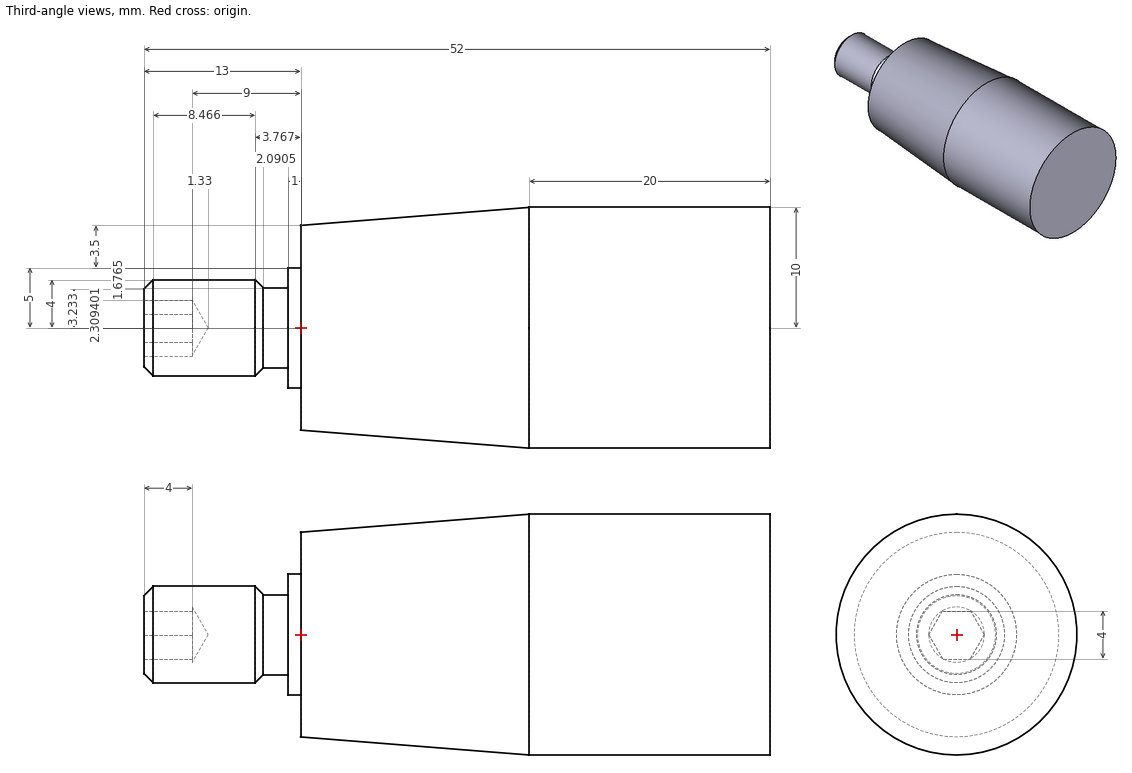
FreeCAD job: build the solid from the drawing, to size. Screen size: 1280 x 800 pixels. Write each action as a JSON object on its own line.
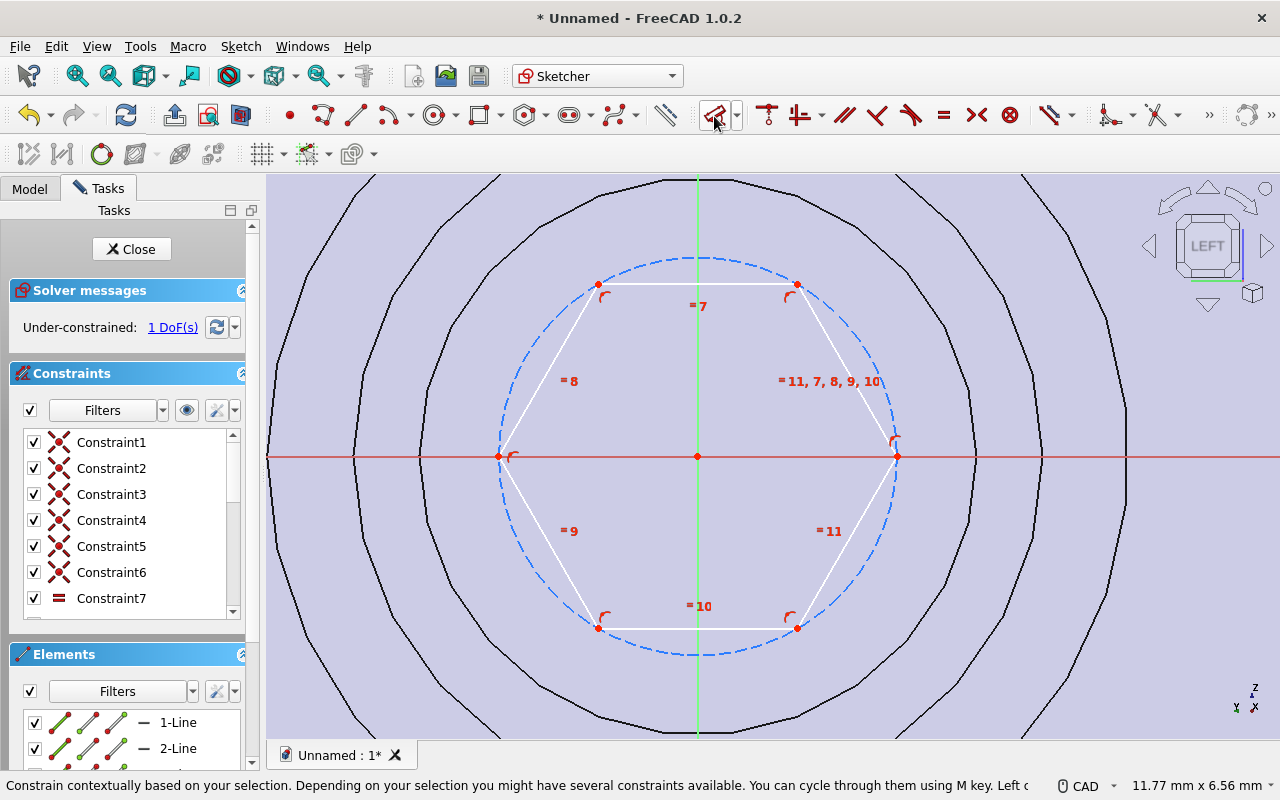
{"action": "left_click", "coordinate": [598, 629]}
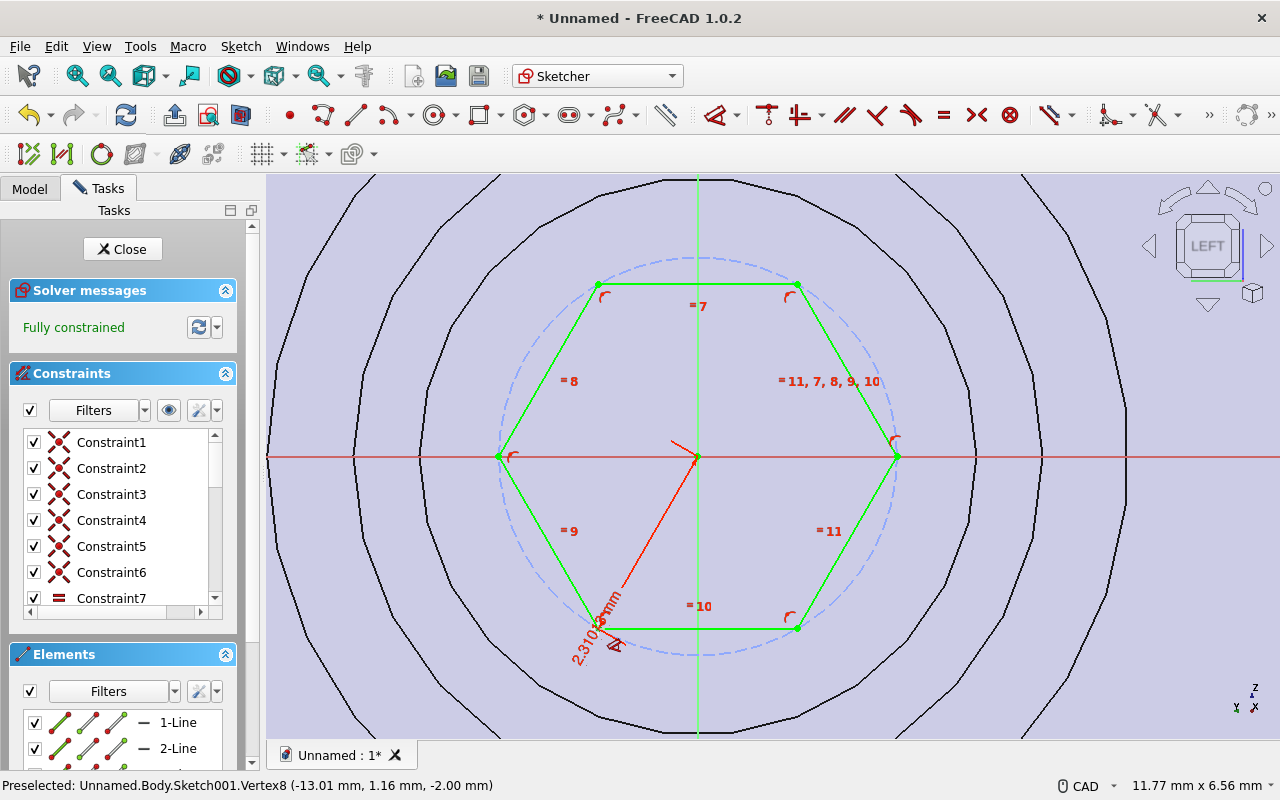
{"action": "left_click", "coordinate": [797, 284]}
{"action": "left_click", "coordinate": [564, 377]}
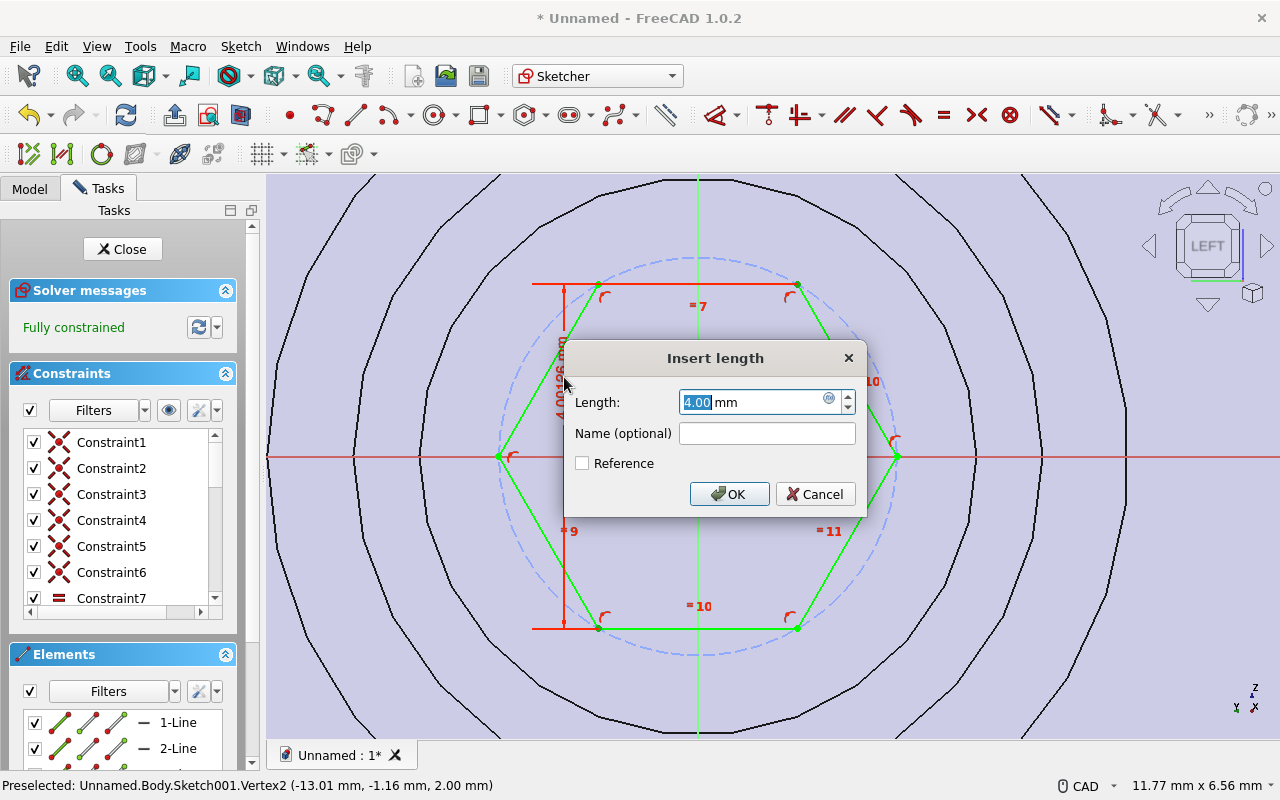
{"action": "type", "text": "4"}
{"action": "key", "text": "Return"}
{"action": "key", "text": "Escape"}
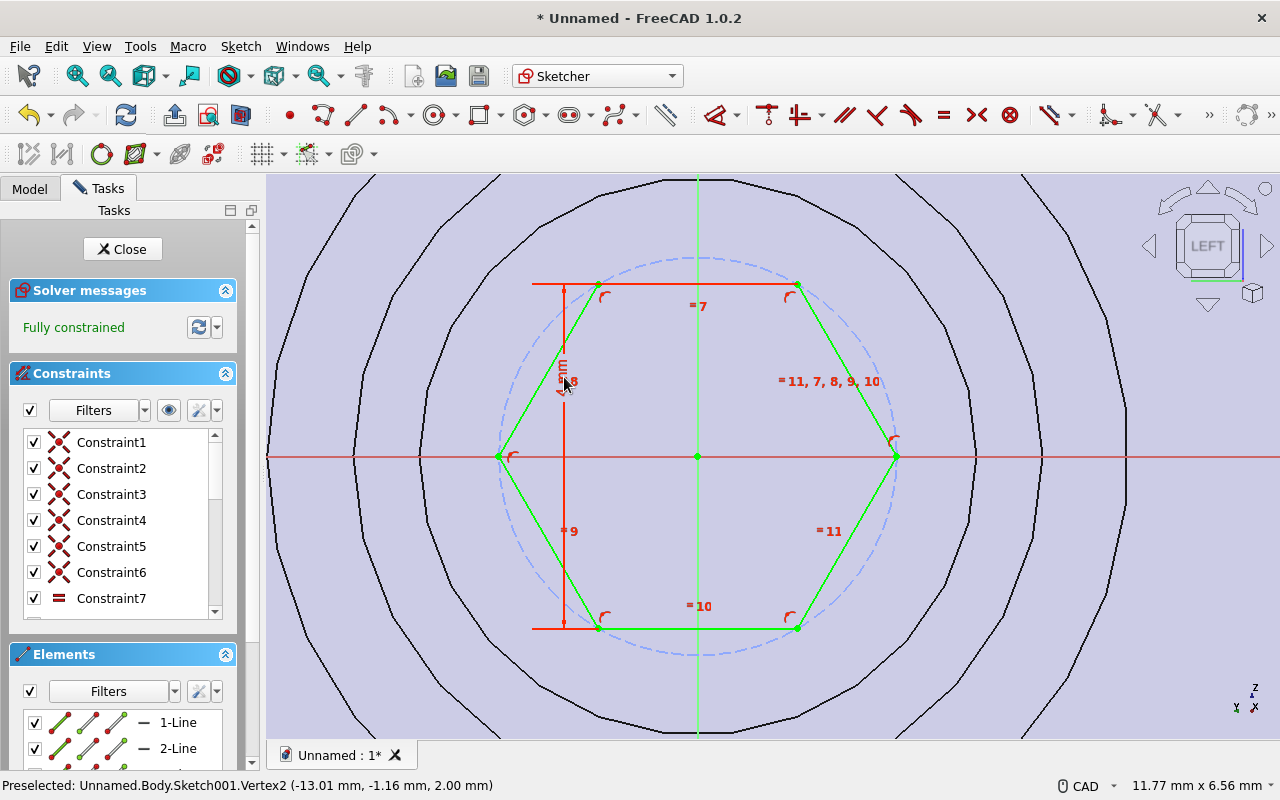
{"action": "left_click", "coordinate": [123, 249]}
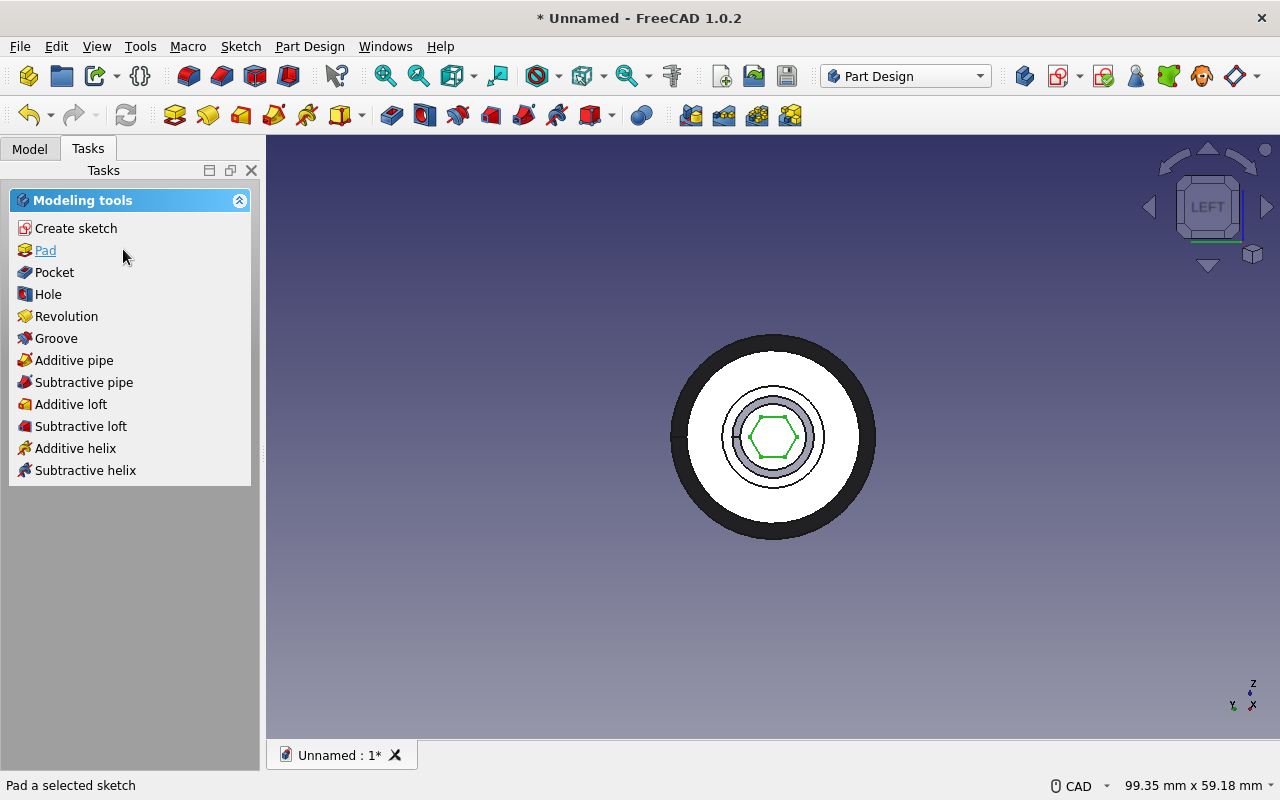
{"action": "left_click", "coordinate": [392, 116]}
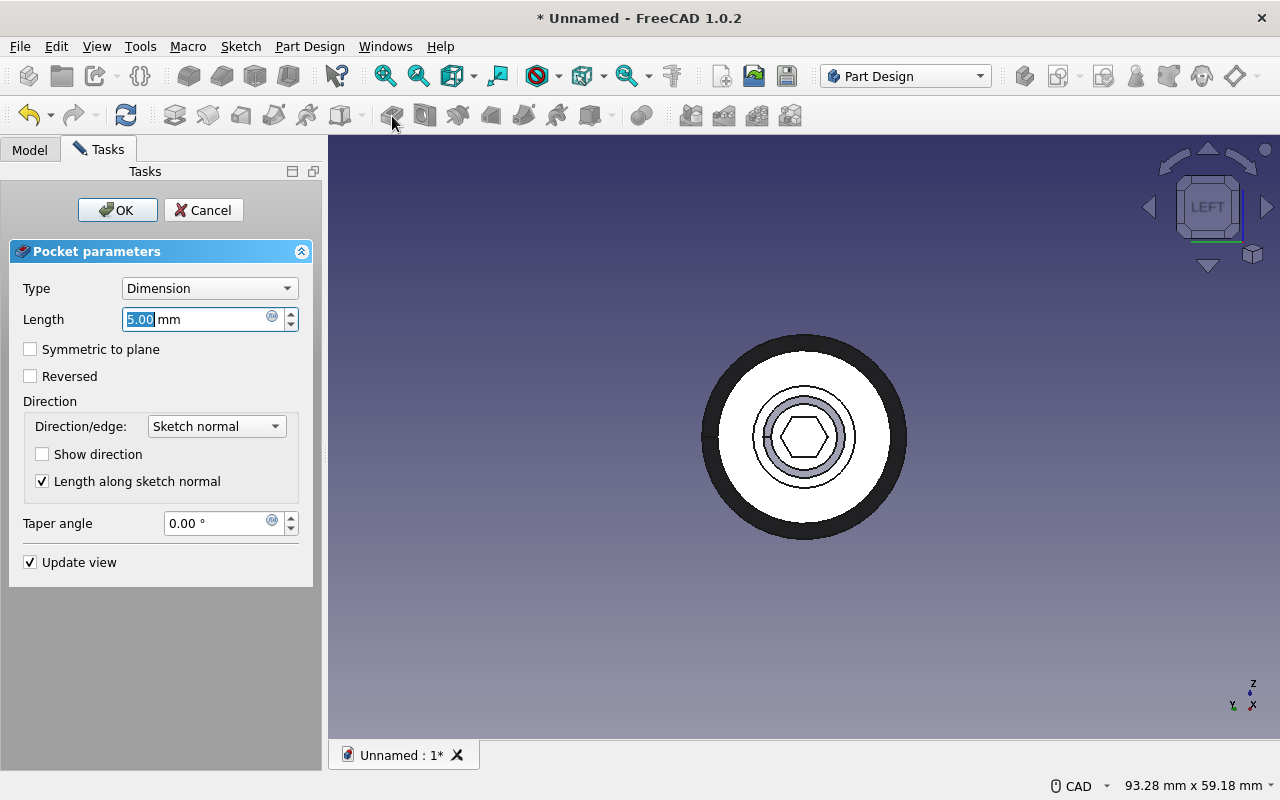
{"action": "type", "text": "4"}
{"action": "key", "text": "Tab"}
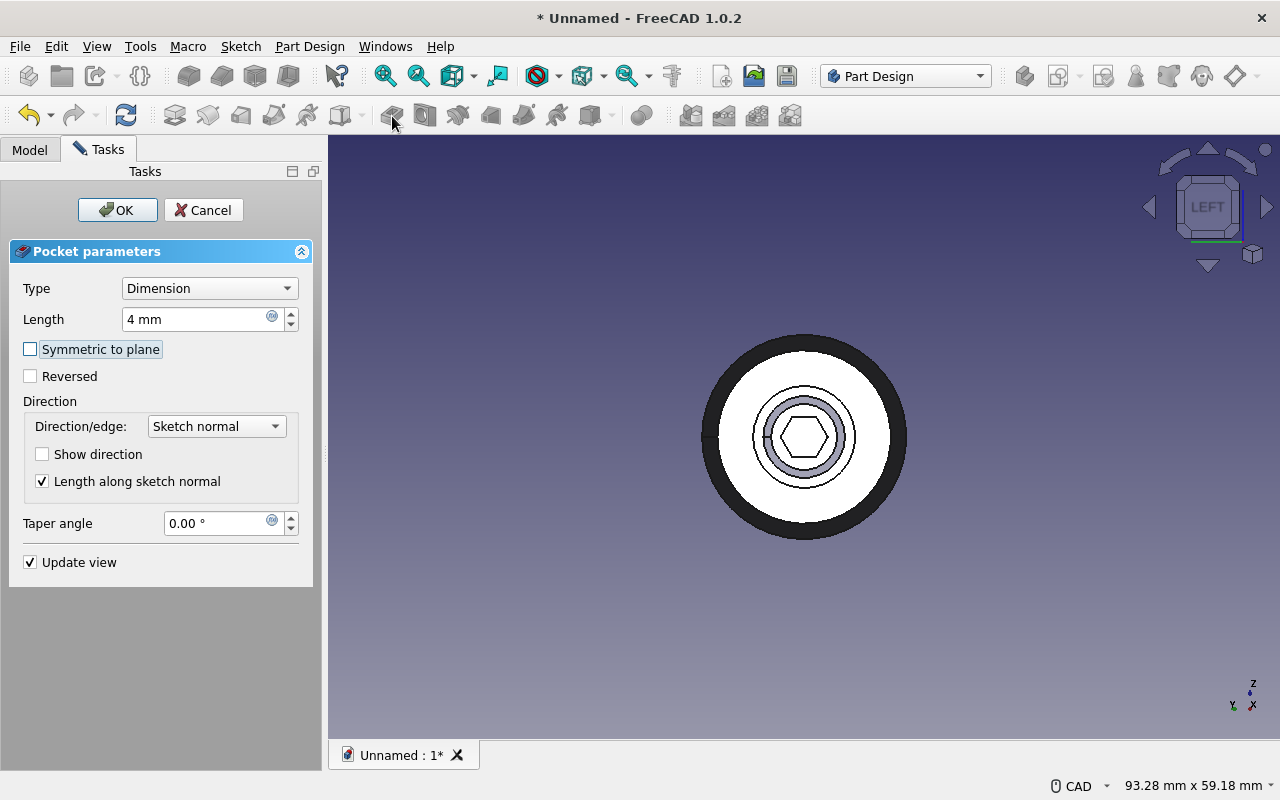
{"action": "left_click", "coordinate": [118, 210]}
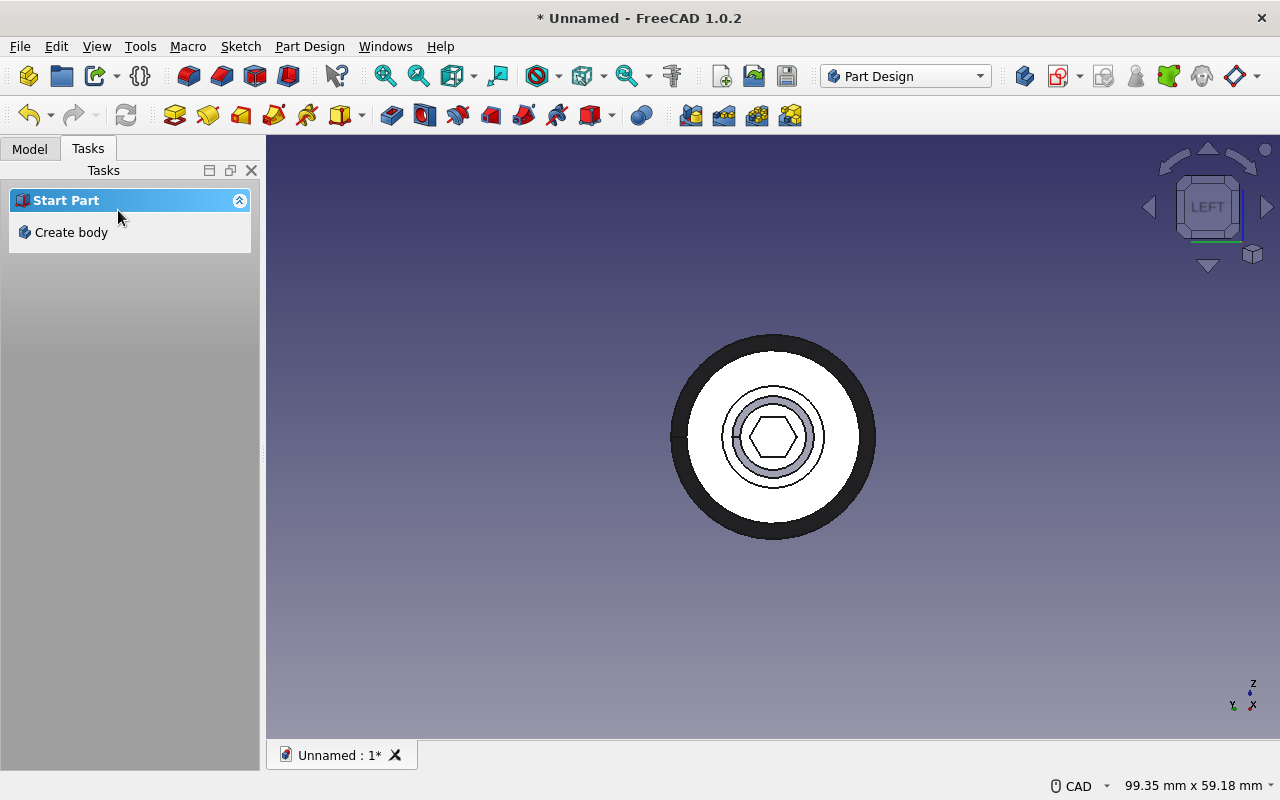
{"action": "key", "text": "v f"}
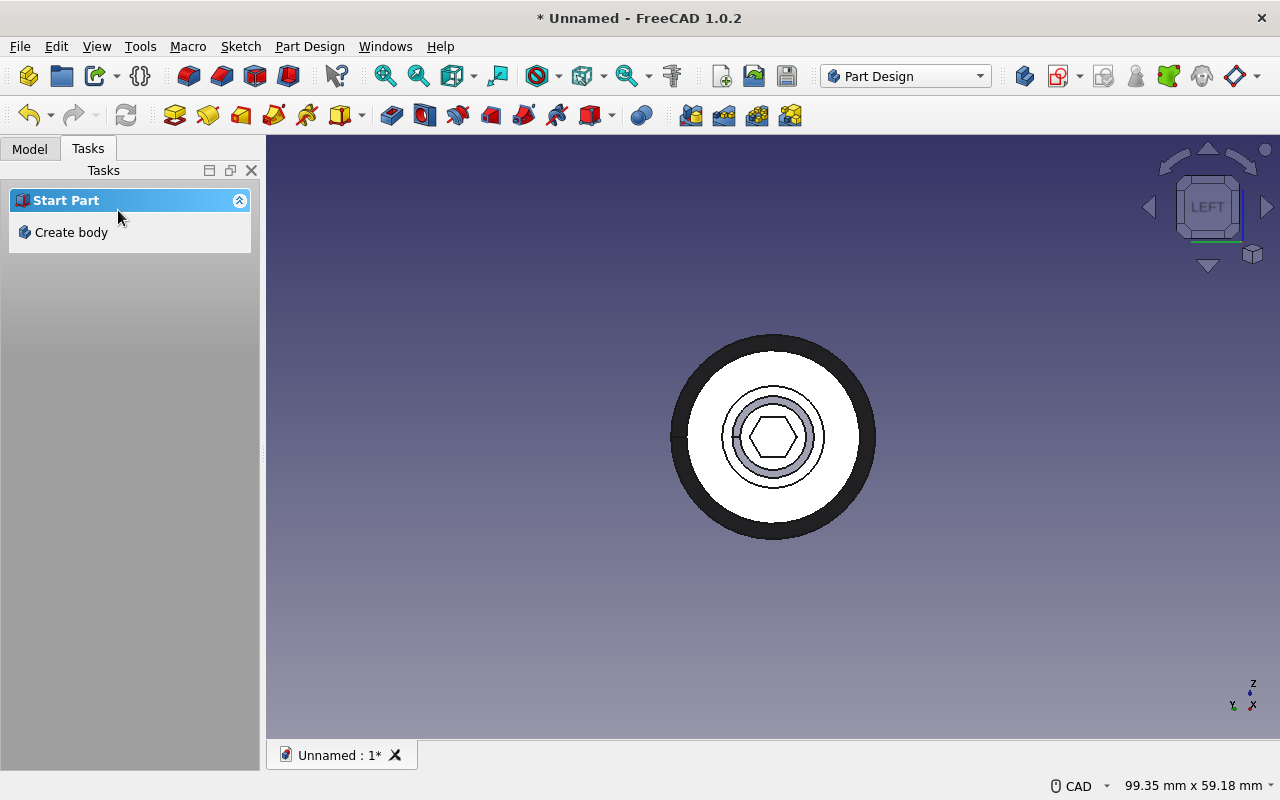
{"action": "left_click", "coordinate": [1058, 76]}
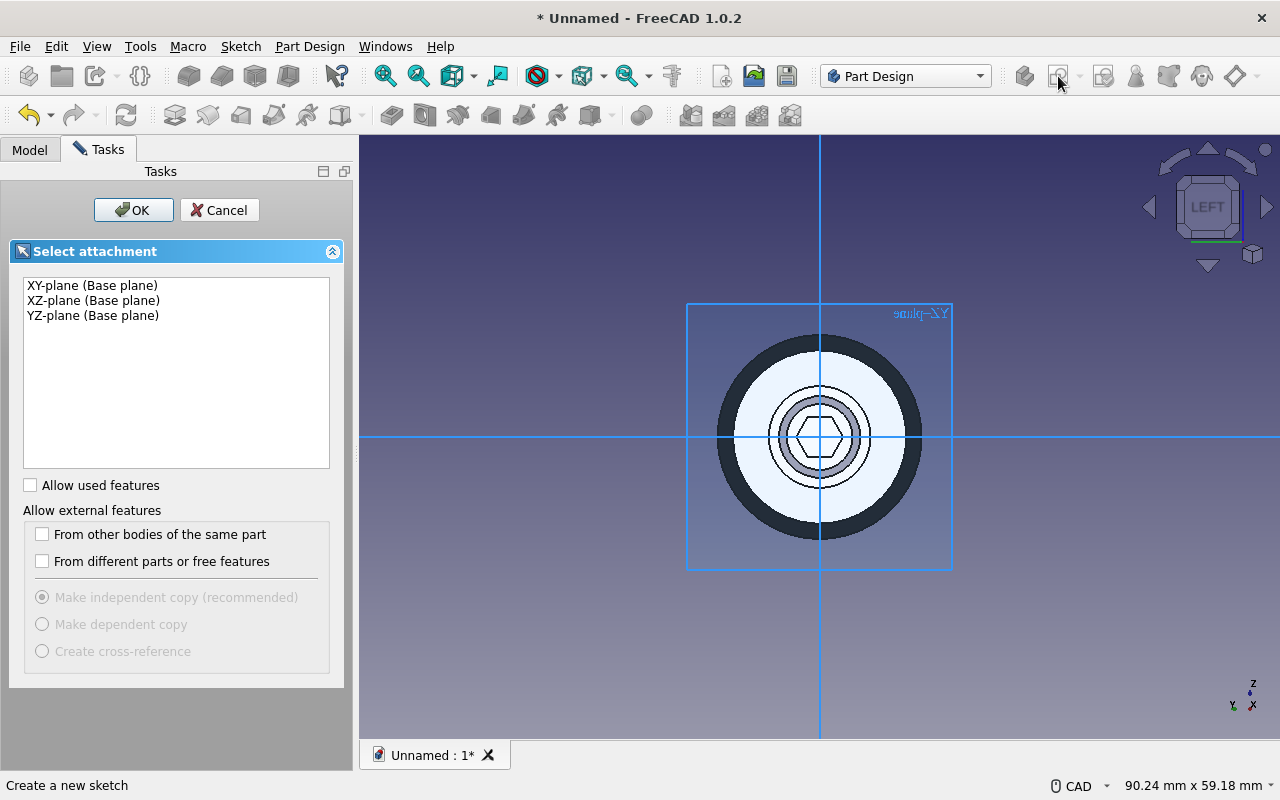
{"action": "left_click", "coordinate": [84, 286]}